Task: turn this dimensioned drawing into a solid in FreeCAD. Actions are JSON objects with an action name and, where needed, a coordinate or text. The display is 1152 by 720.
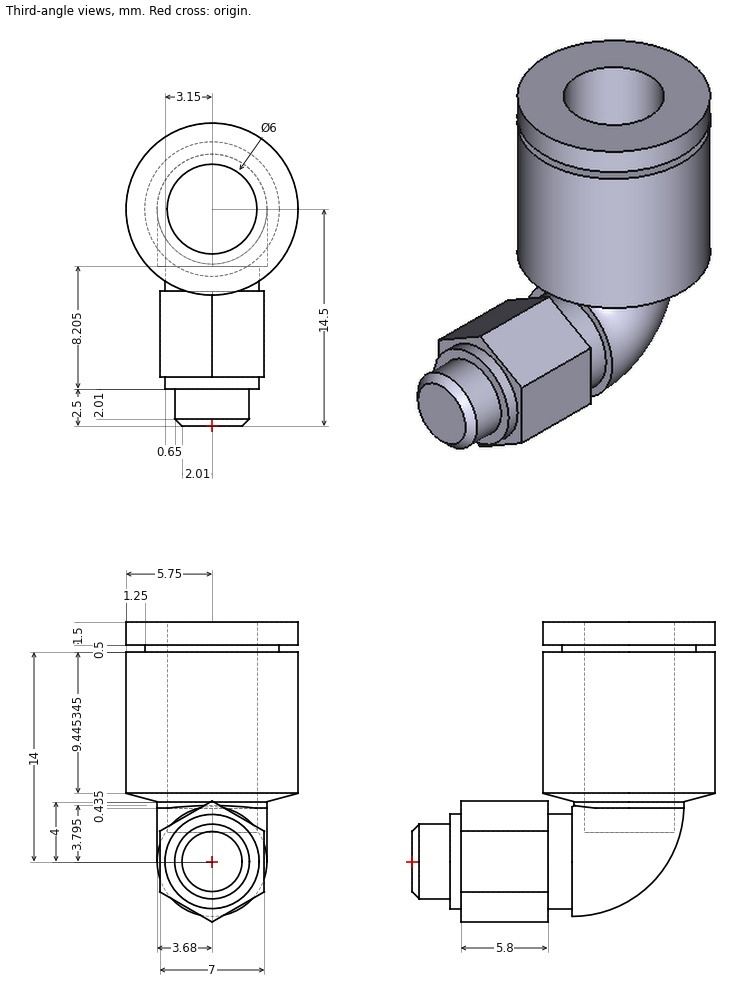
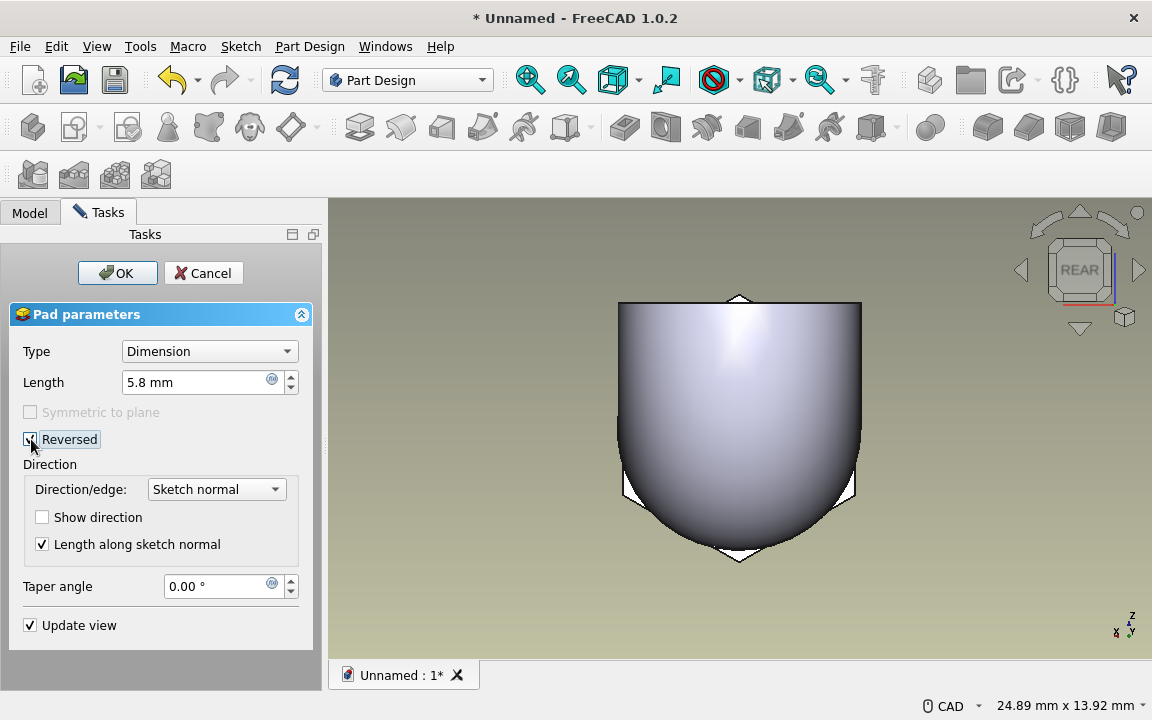
{"action": "left_click", "coordinate": [118, 273]}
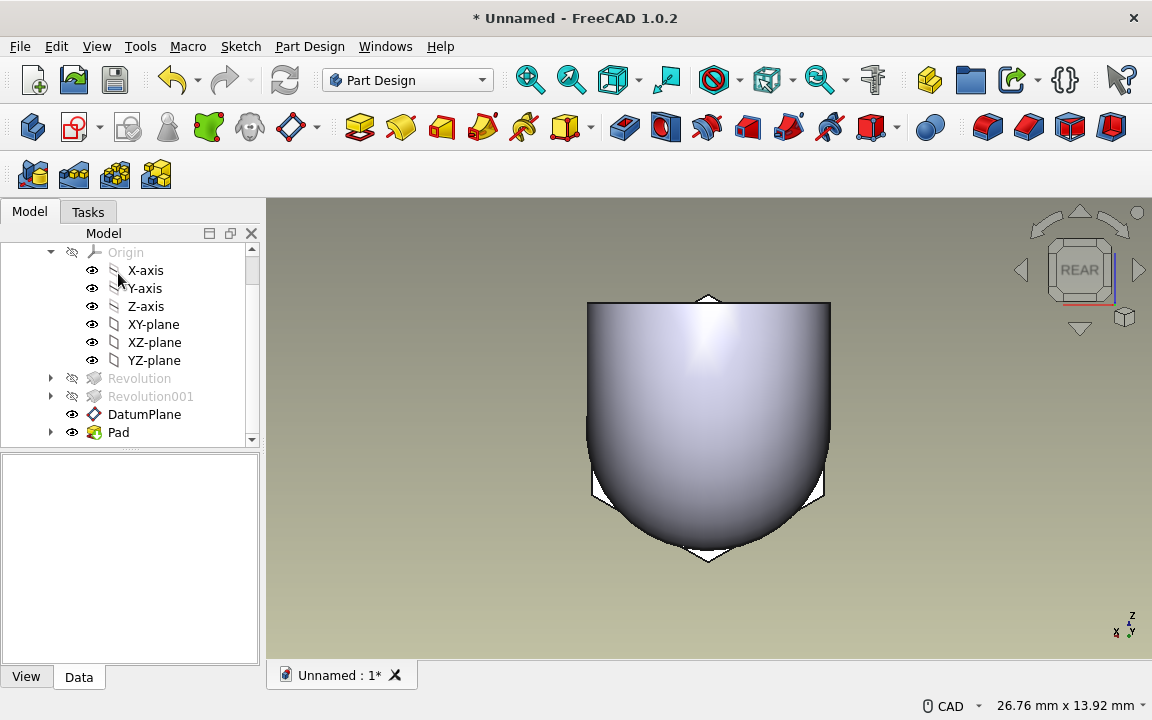
{"action": "left_click", "coordinate": [117, 414]}
{"action": "key", "text": "space"}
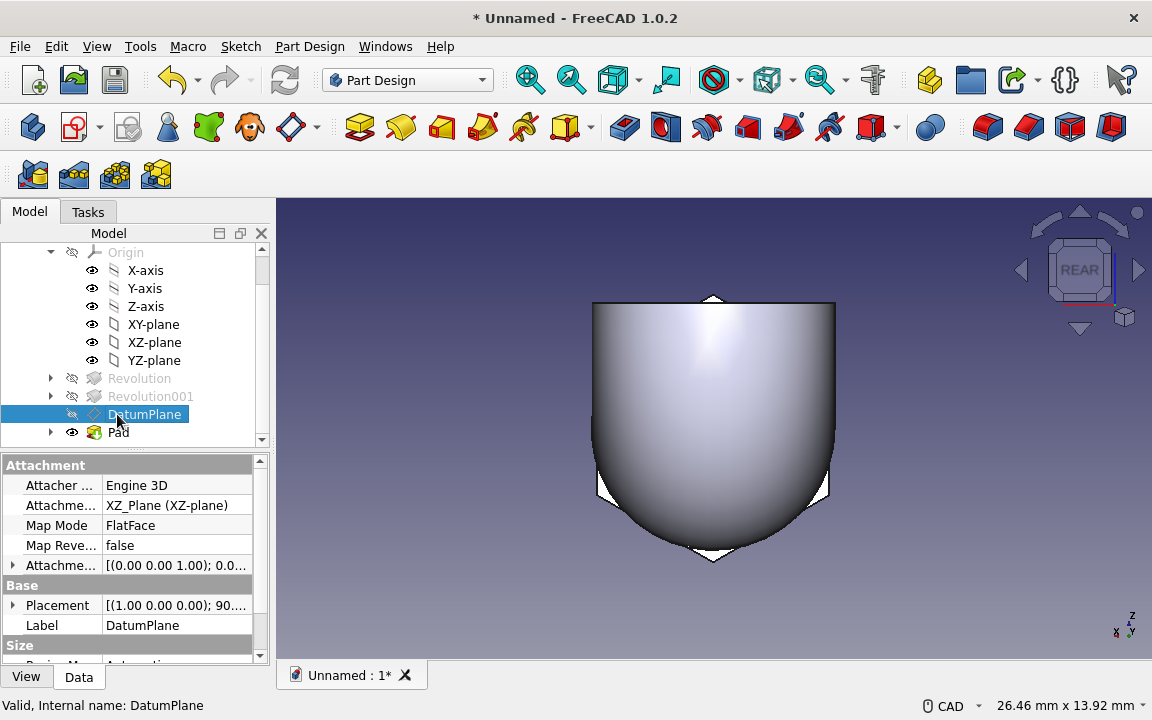
{"action": "left_click", "coordinate": [137, 342]}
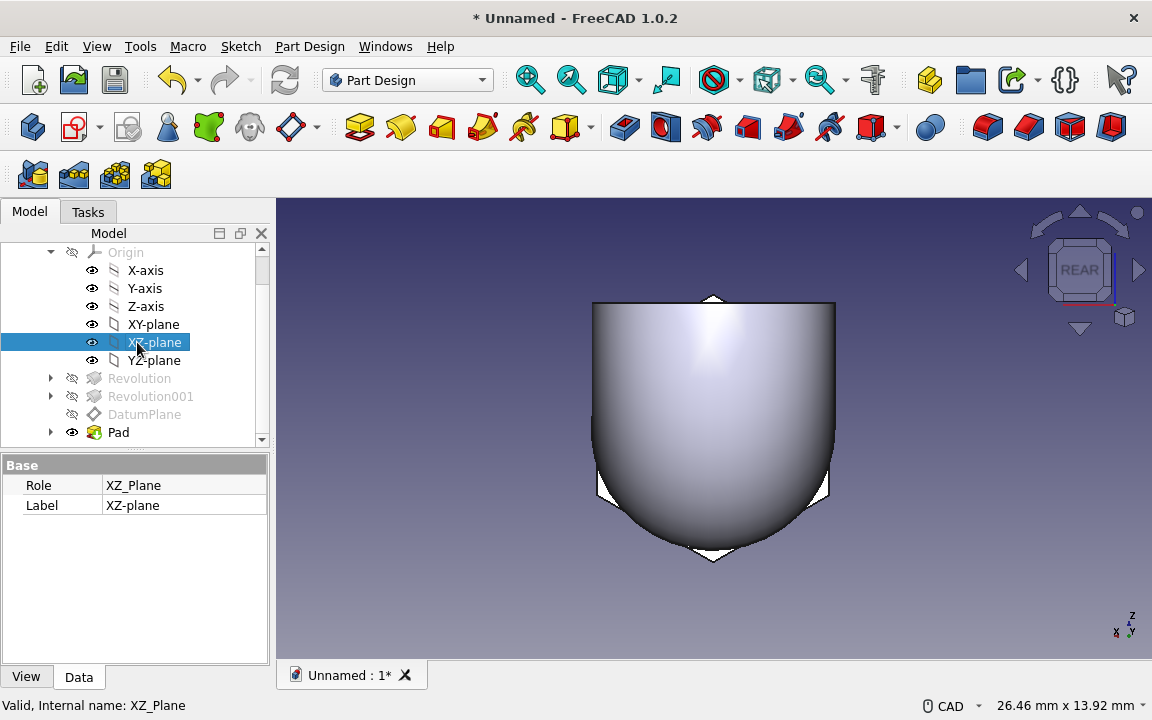
{"action": "left_click", "coordinate": [290, 128]}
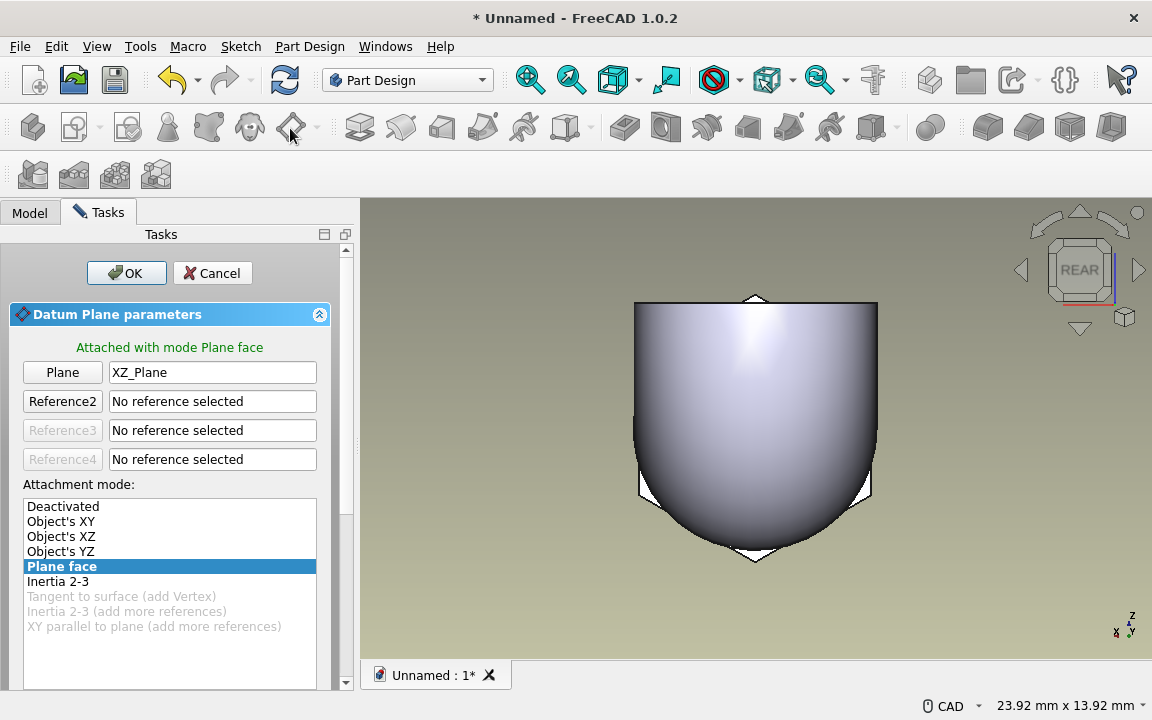
{"action": "scroll", "coordinate": [346, 467], "scroll_direction": "down", "scroll_amount": 4}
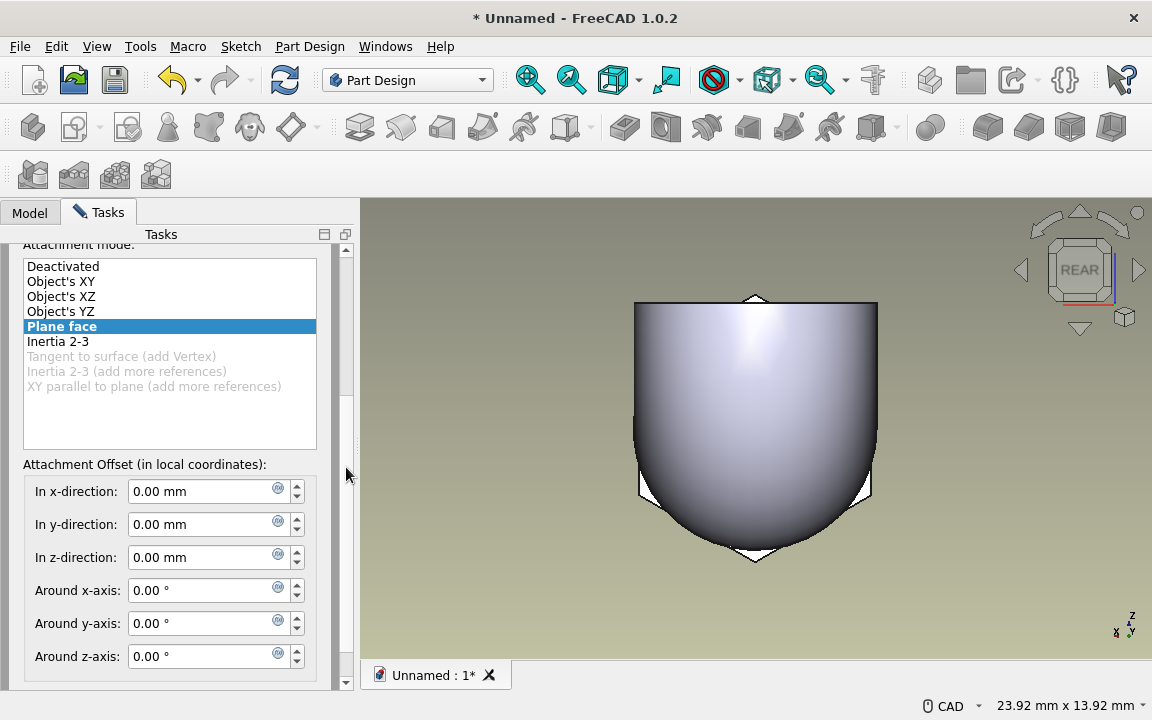
{"action": "triple_click", "coordinate": [210, 558]}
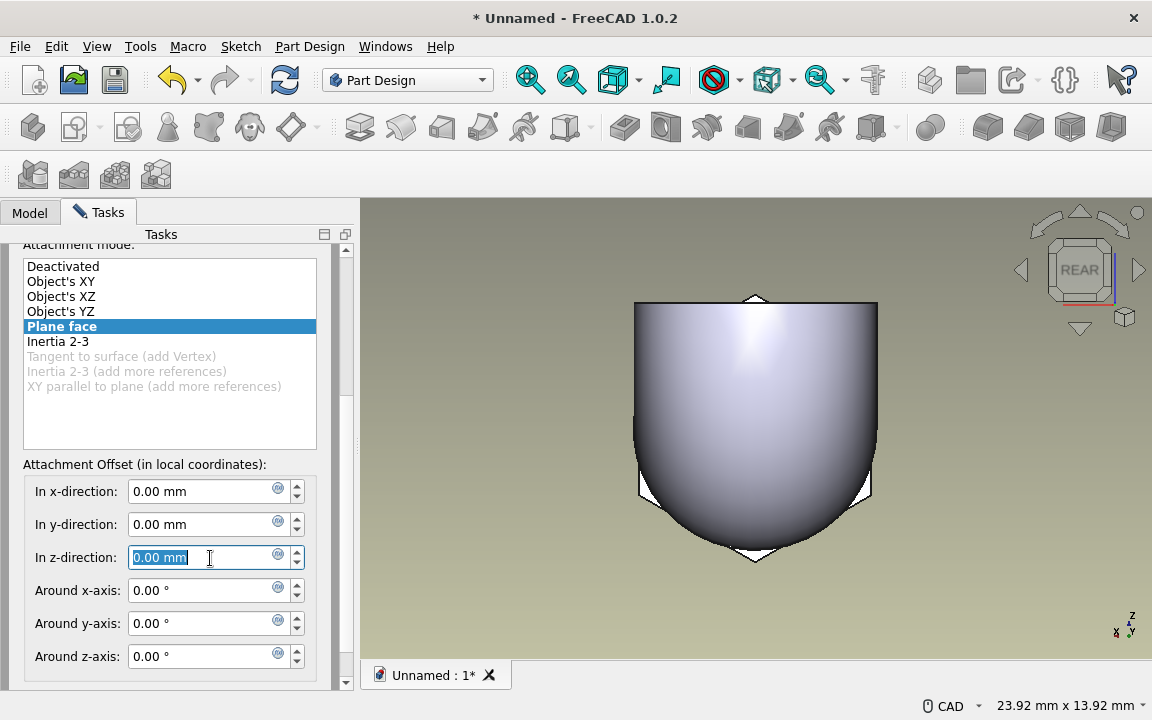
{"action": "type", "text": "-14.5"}
{"action": "key", "text": "Tab"}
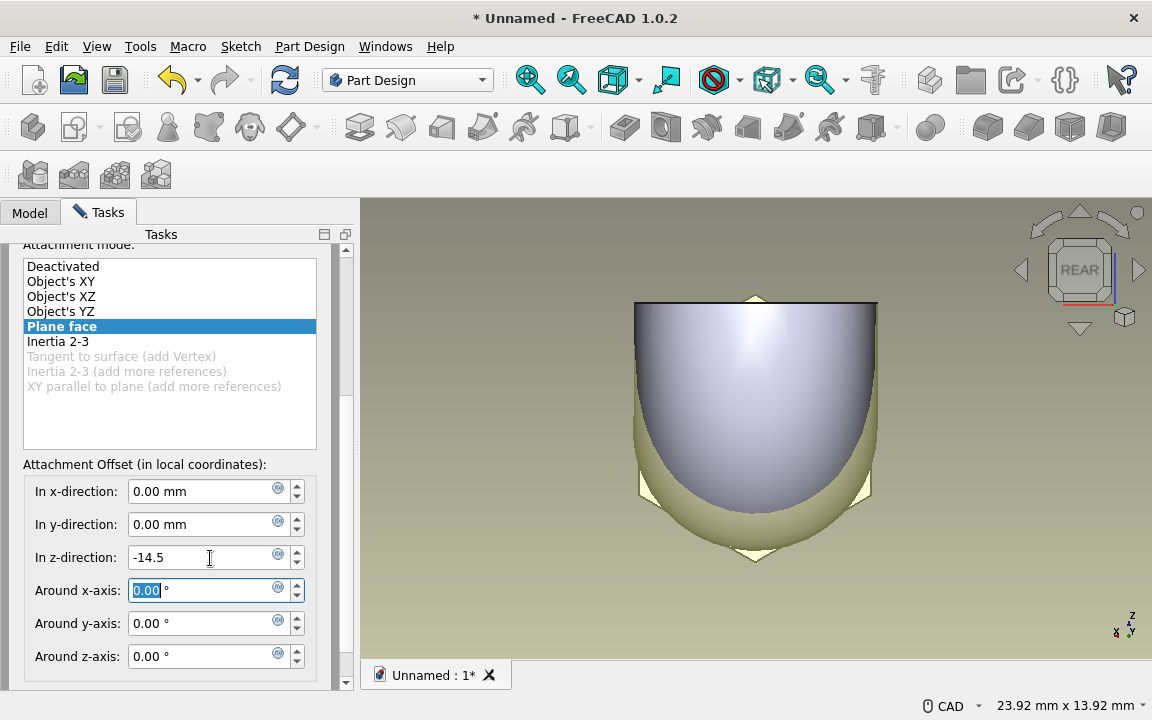
{"action": "scroll", "coordinate": [346, 467], "scroll_direction": "up", "scroll_amount": 5}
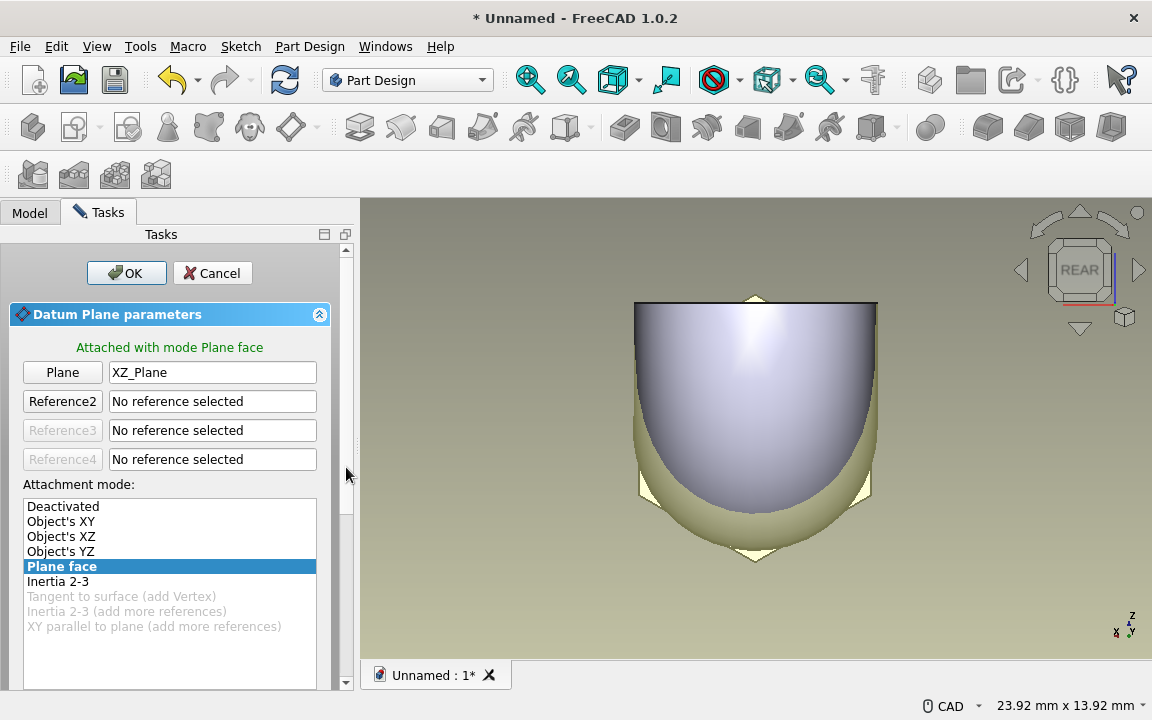
{"action": "left_click", "coordinate": [127, 273]}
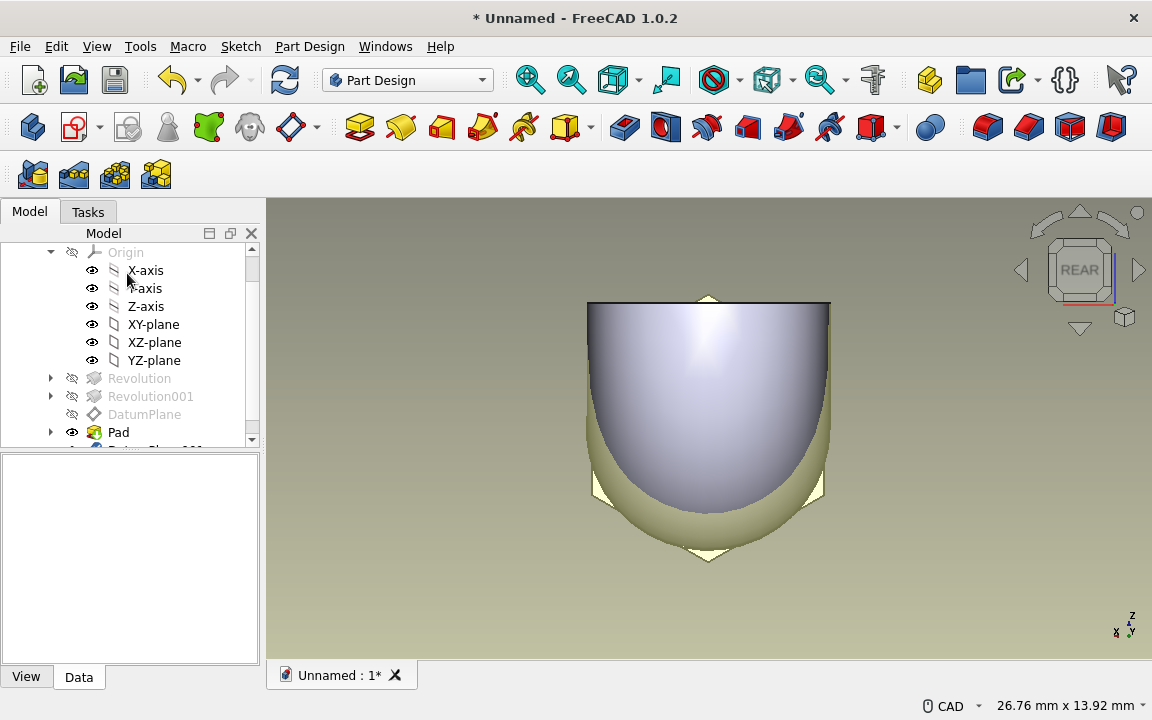
{"action": "scroll", "coordinate": [141, 338], "scroll_direction": "down", "scroll_amount": 3}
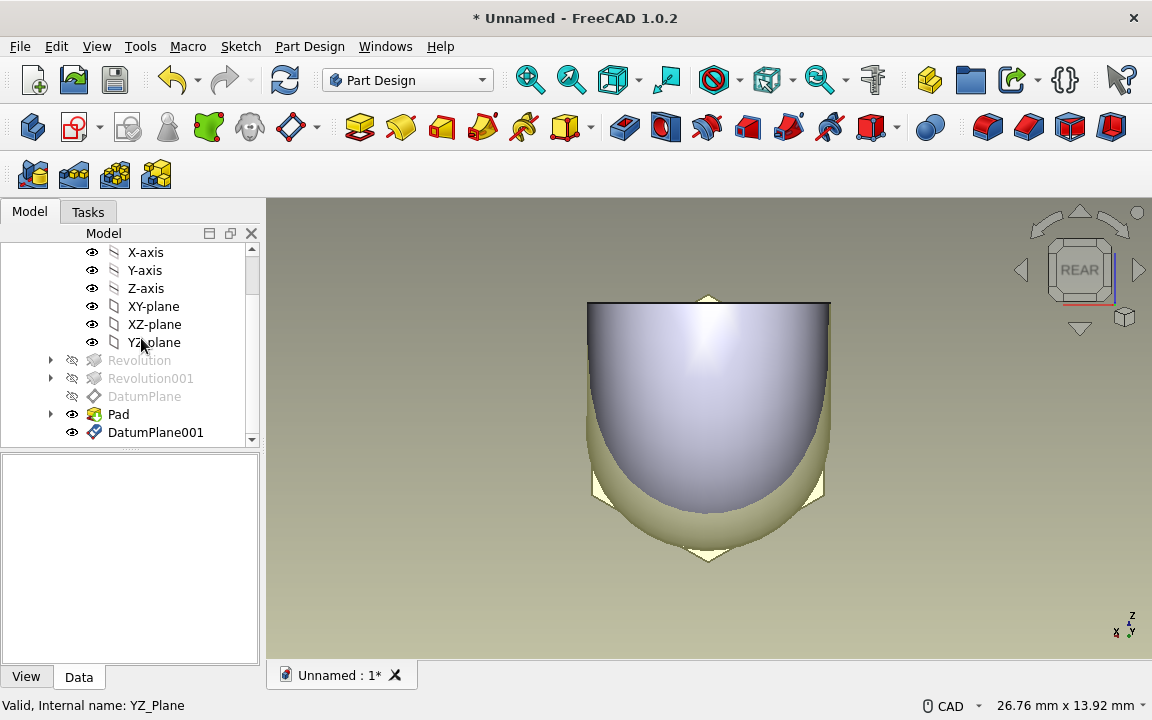
{"action": "left_click", "coordinate": [117, 432]}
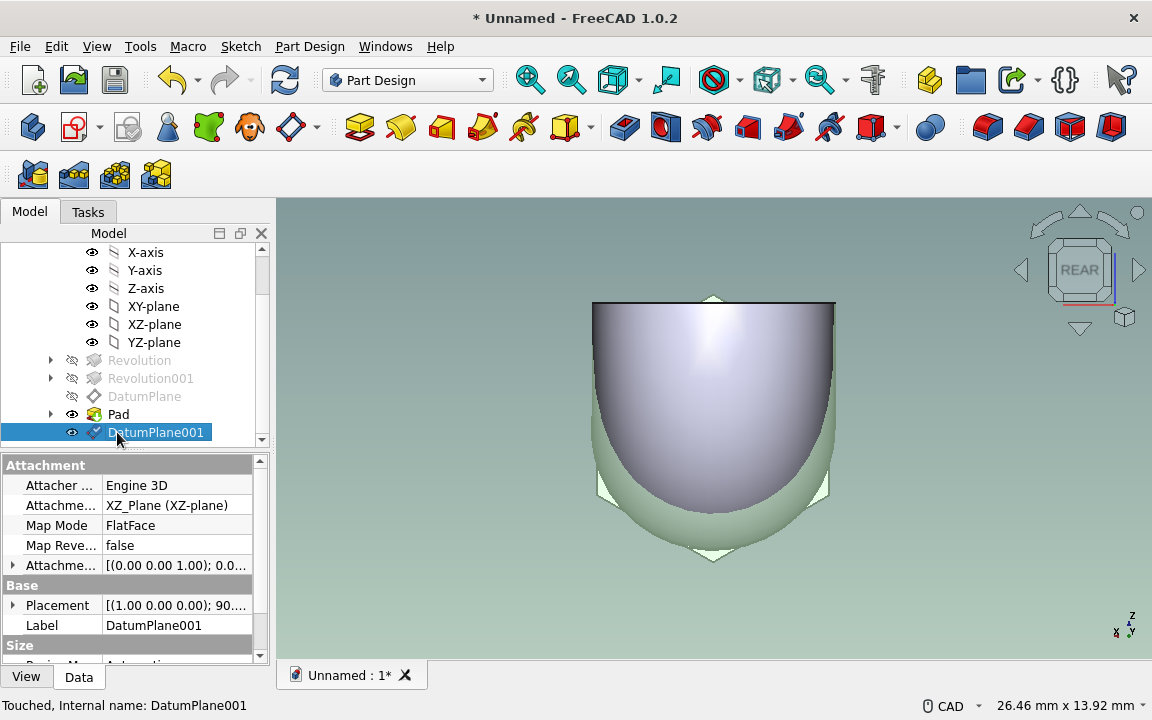
{"action": "left_click", "coordinate": [74, 128]}